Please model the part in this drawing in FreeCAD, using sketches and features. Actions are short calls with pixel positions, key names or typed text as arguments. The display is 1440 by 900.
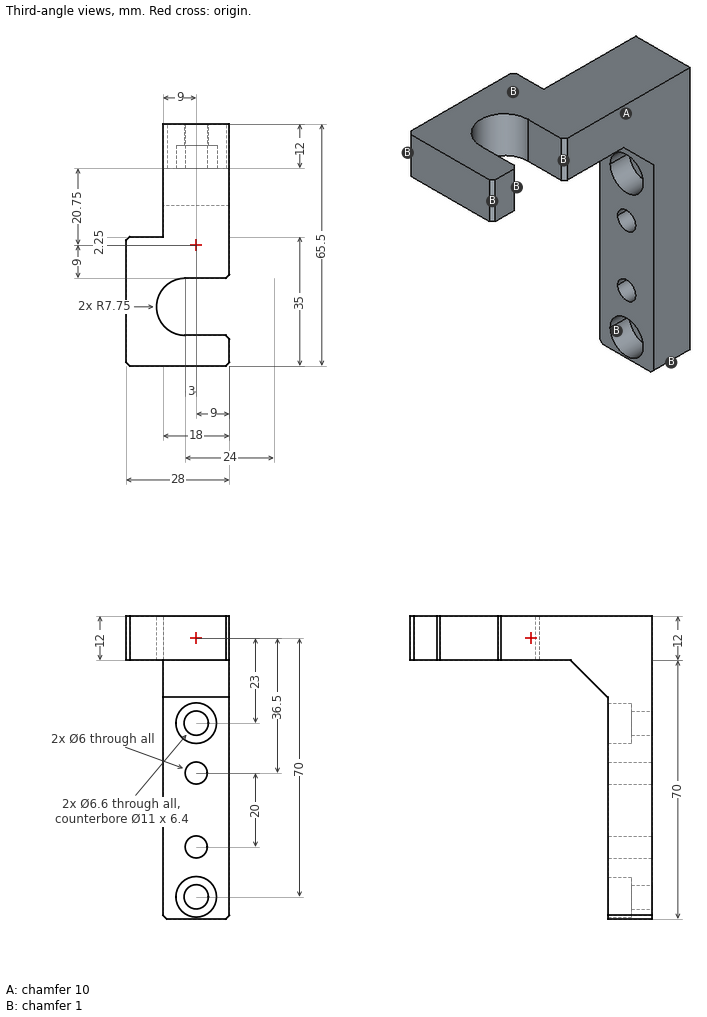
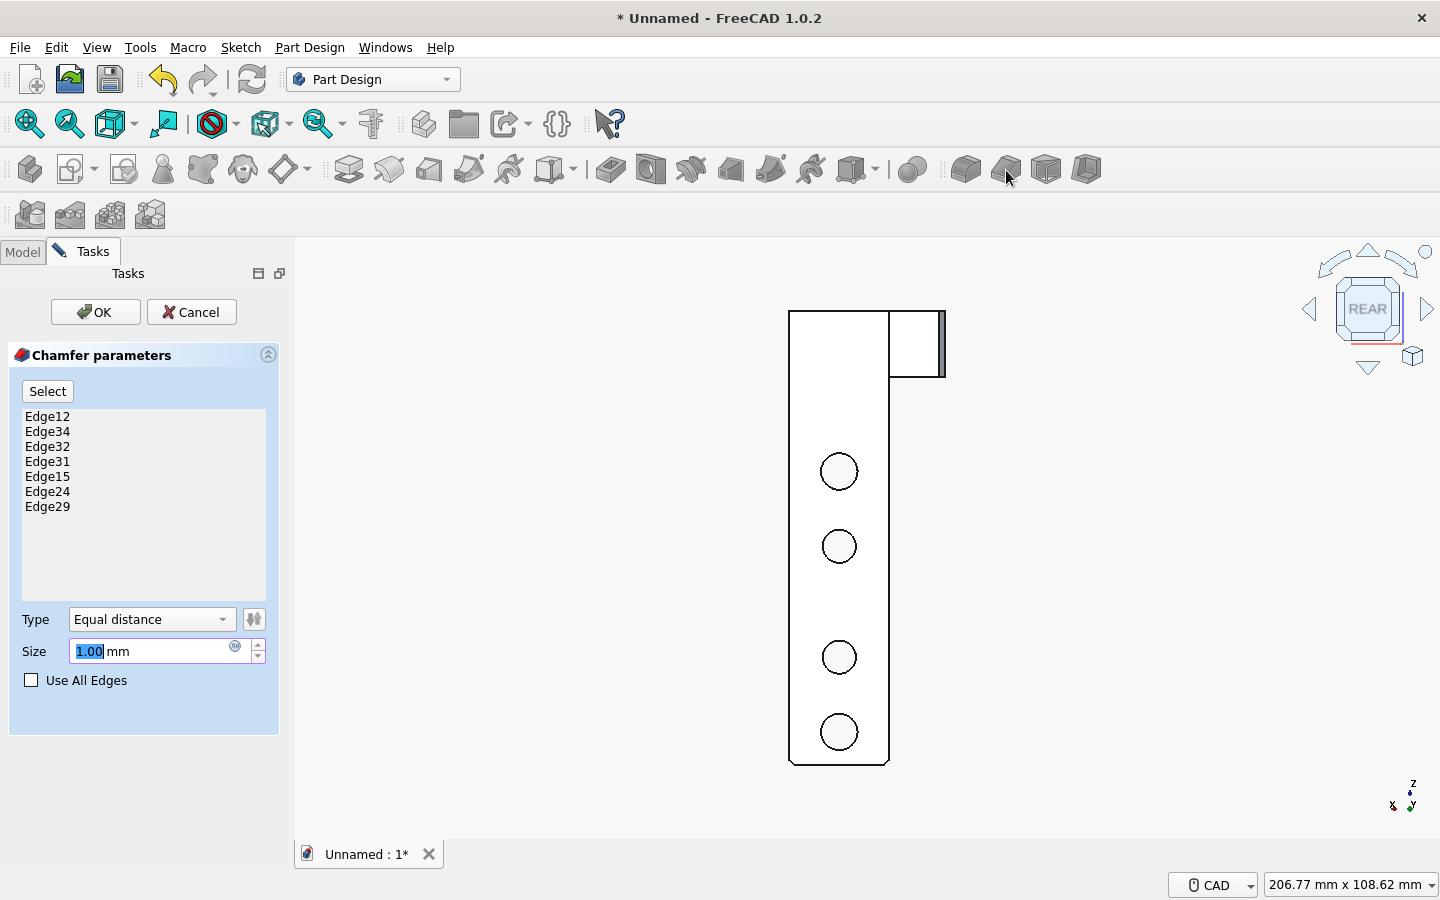
text(1)
key(Tab)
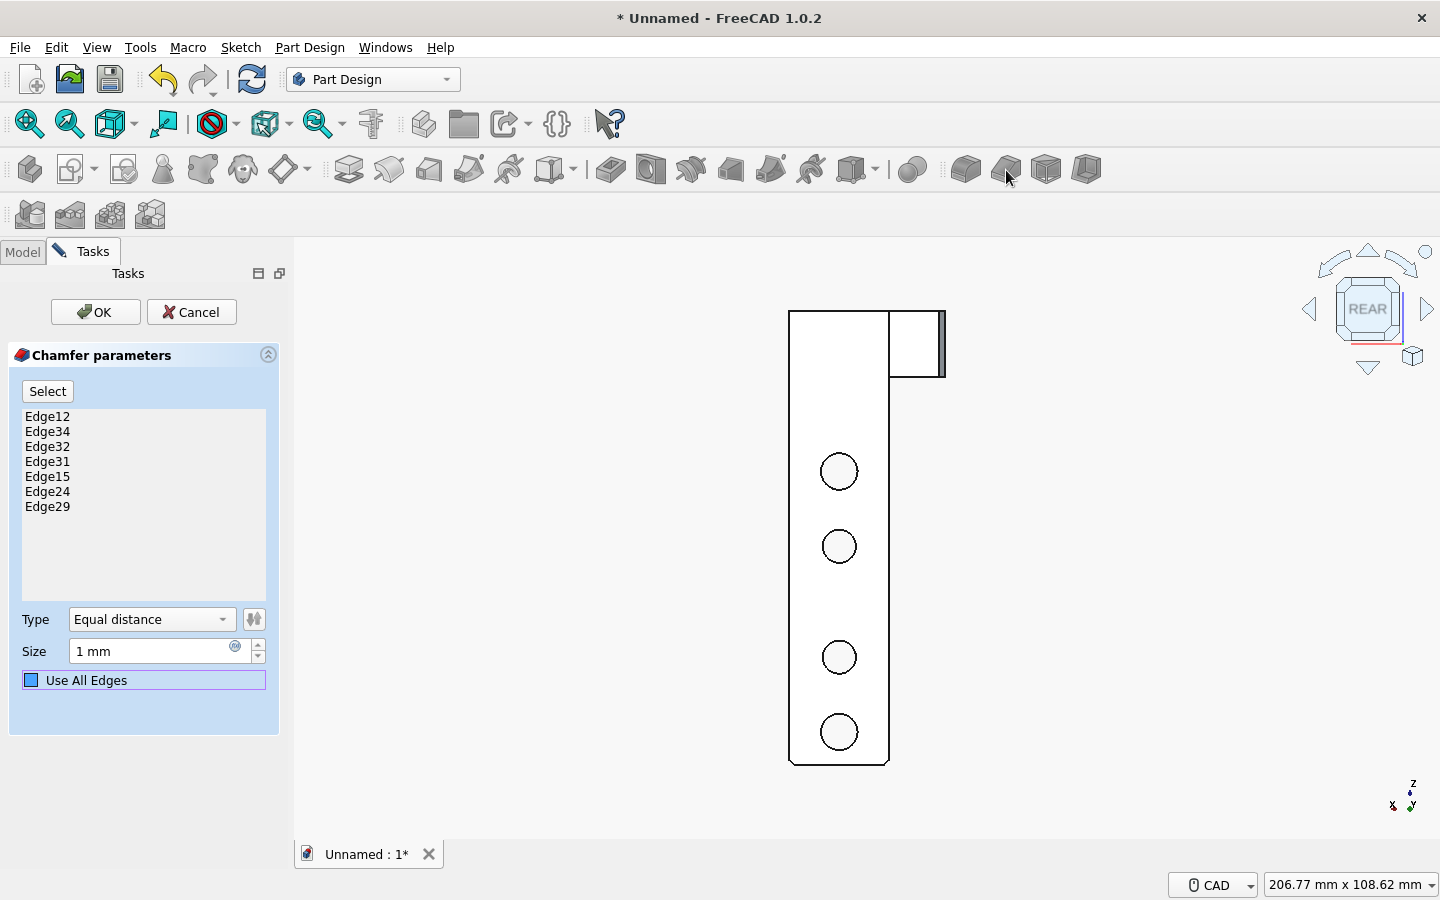
click(96, 312)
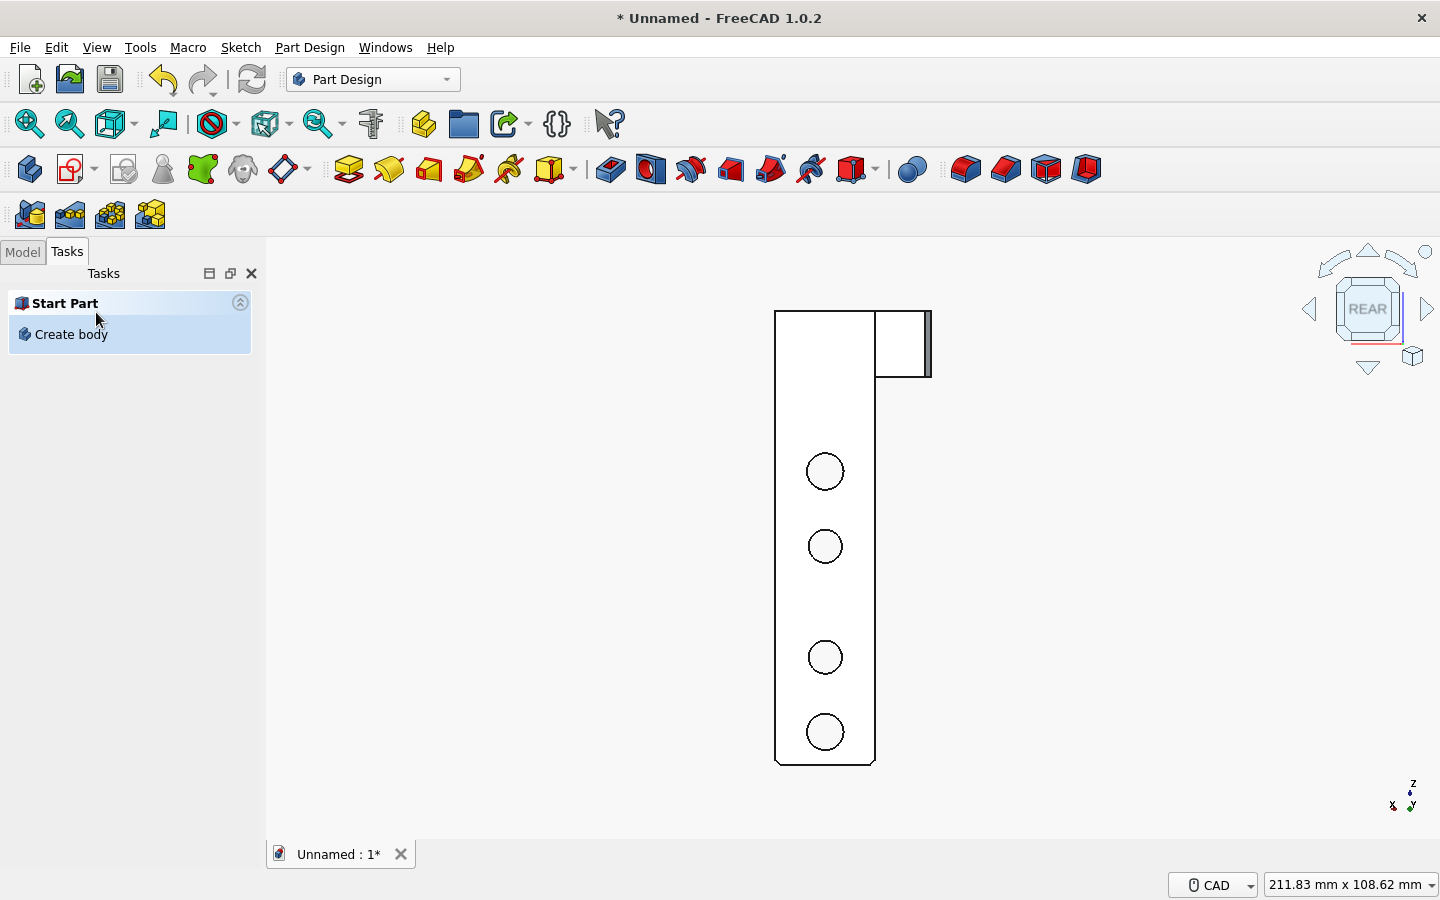
key(0)